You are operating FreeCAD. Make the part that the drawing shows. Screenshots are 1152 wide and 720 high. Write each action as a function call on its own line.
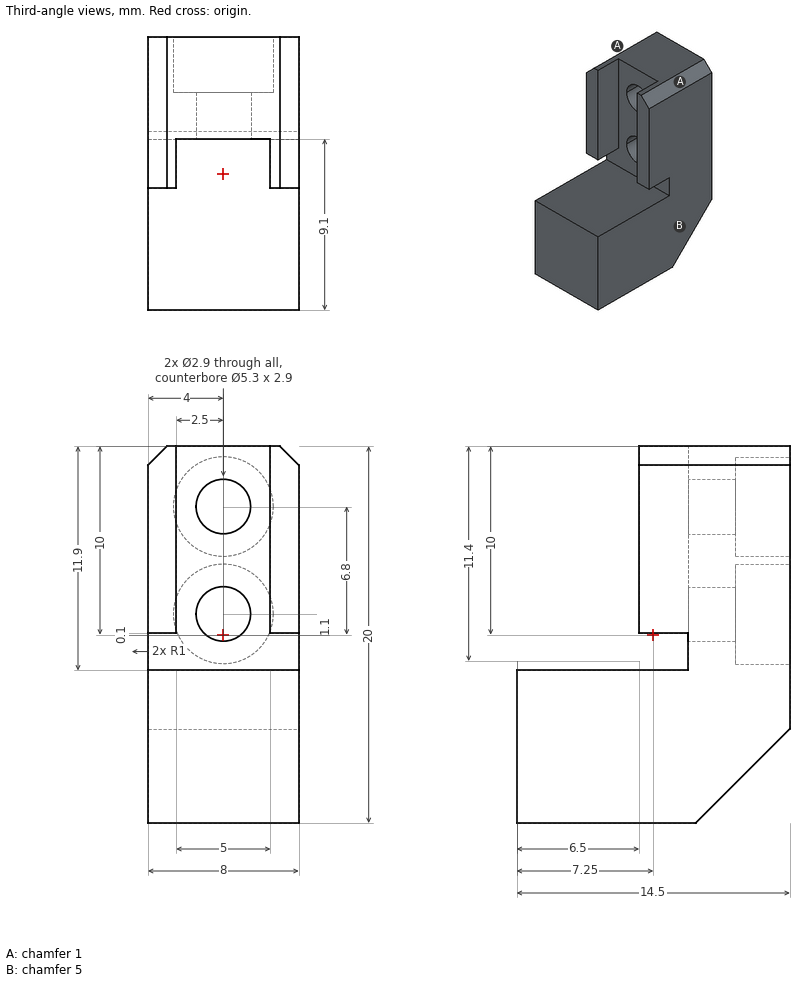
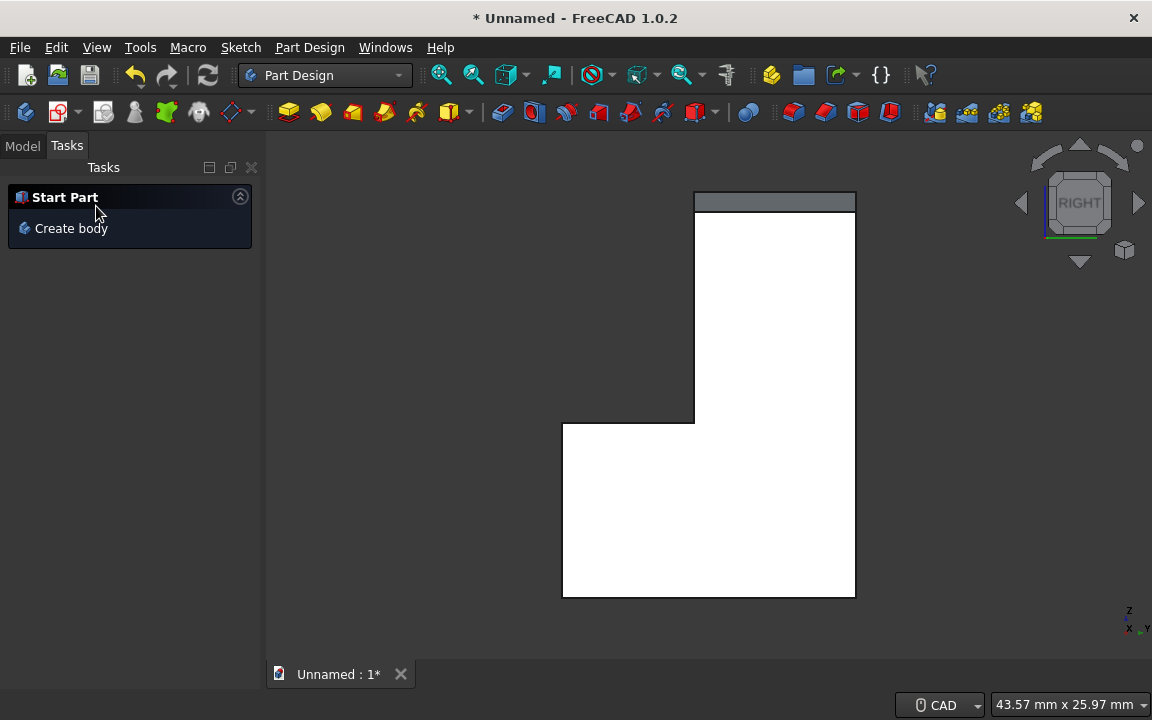
key(5)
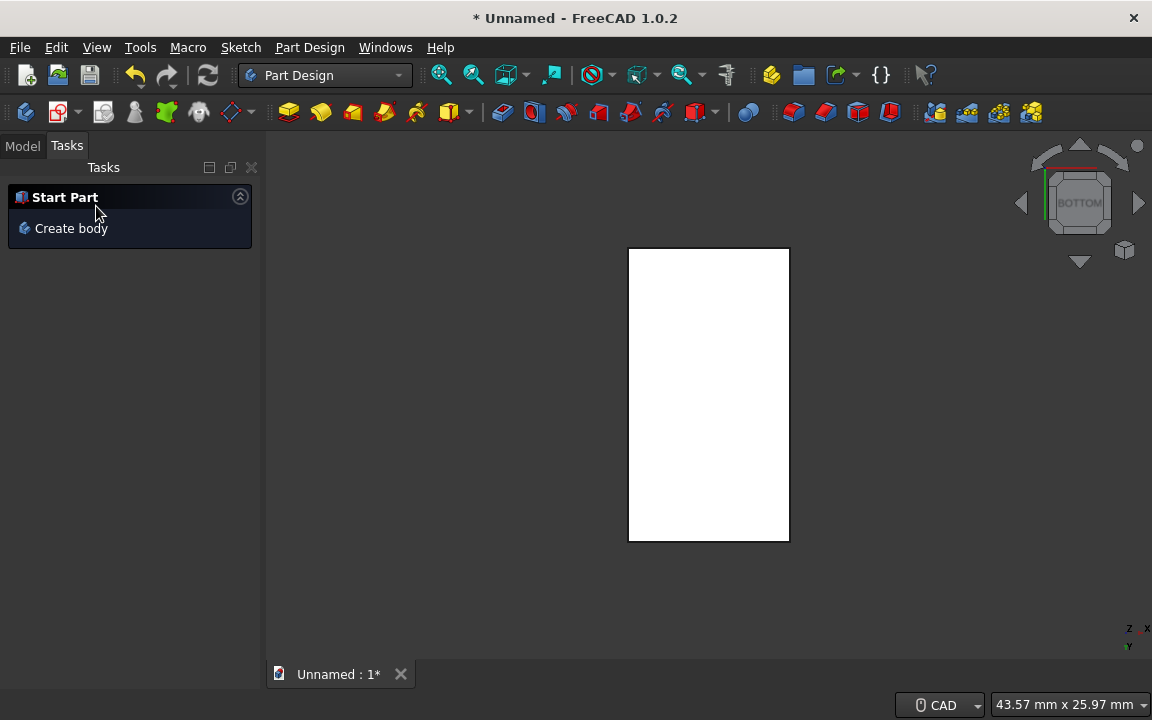
key(4)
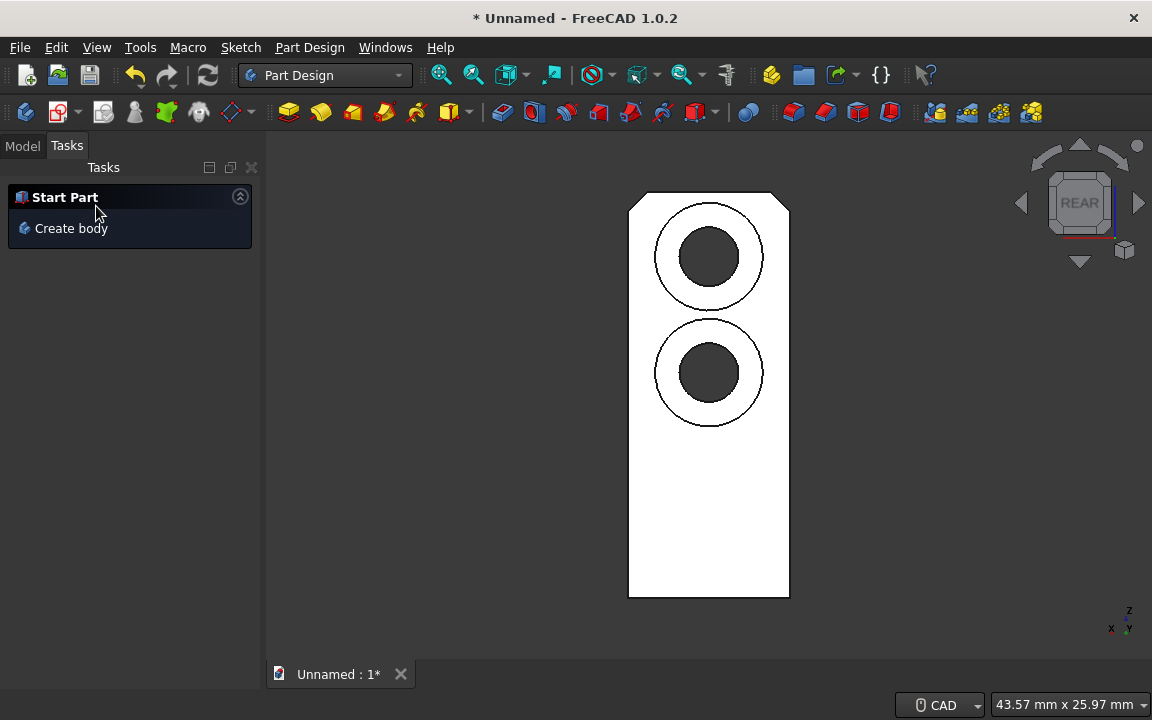
click(709, 597)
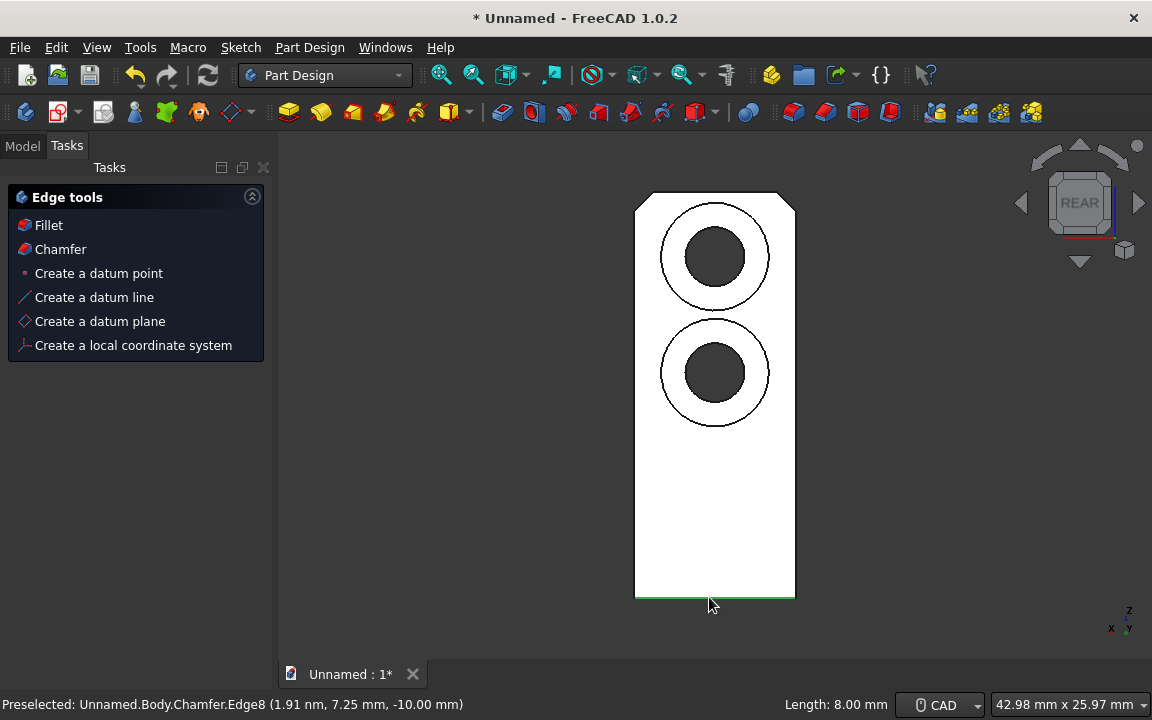
click(826, 112)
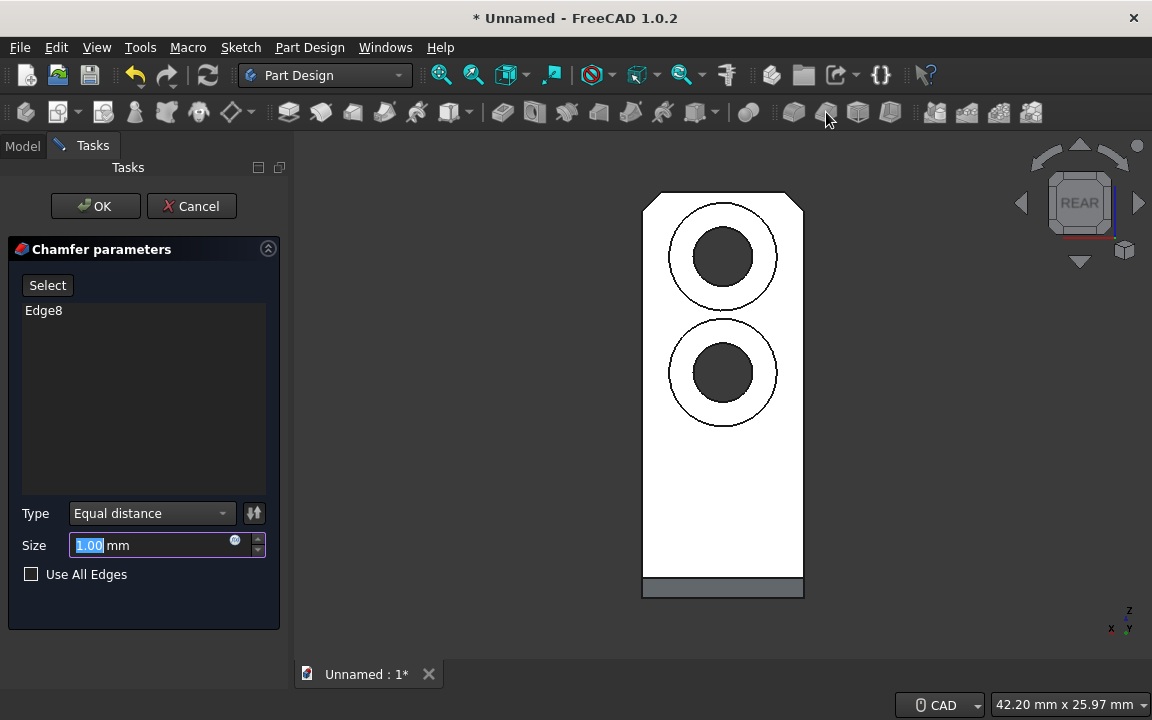
text(5)
key(Tab)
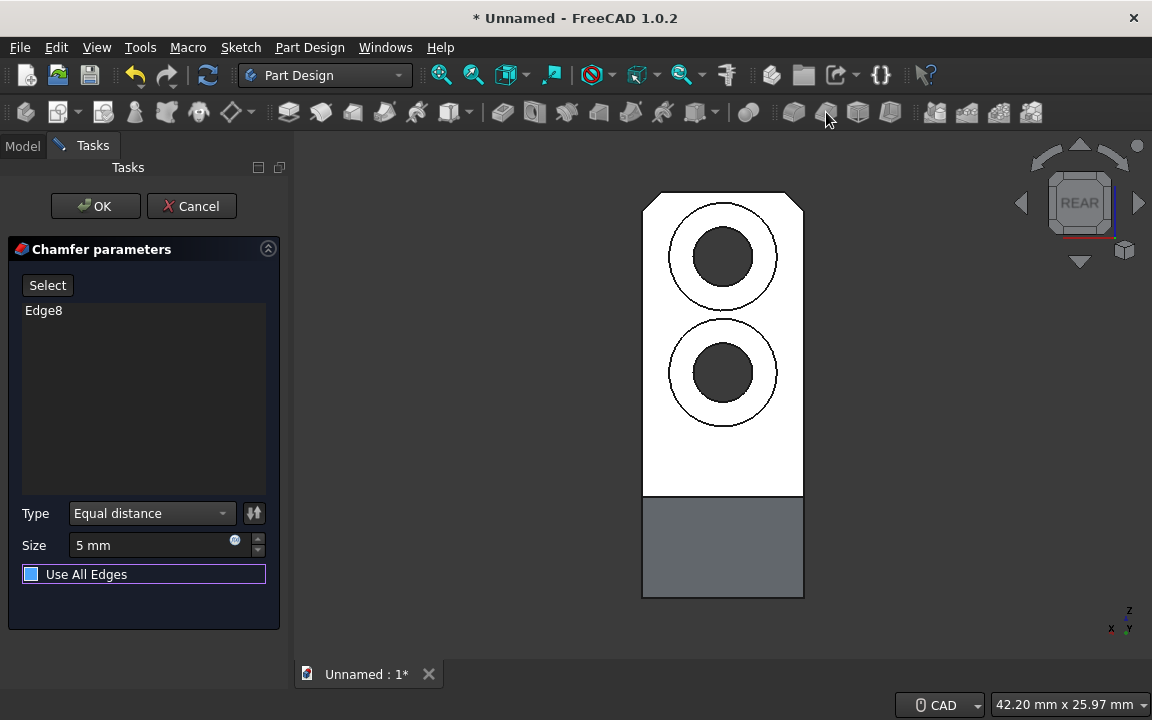
click(96, 206)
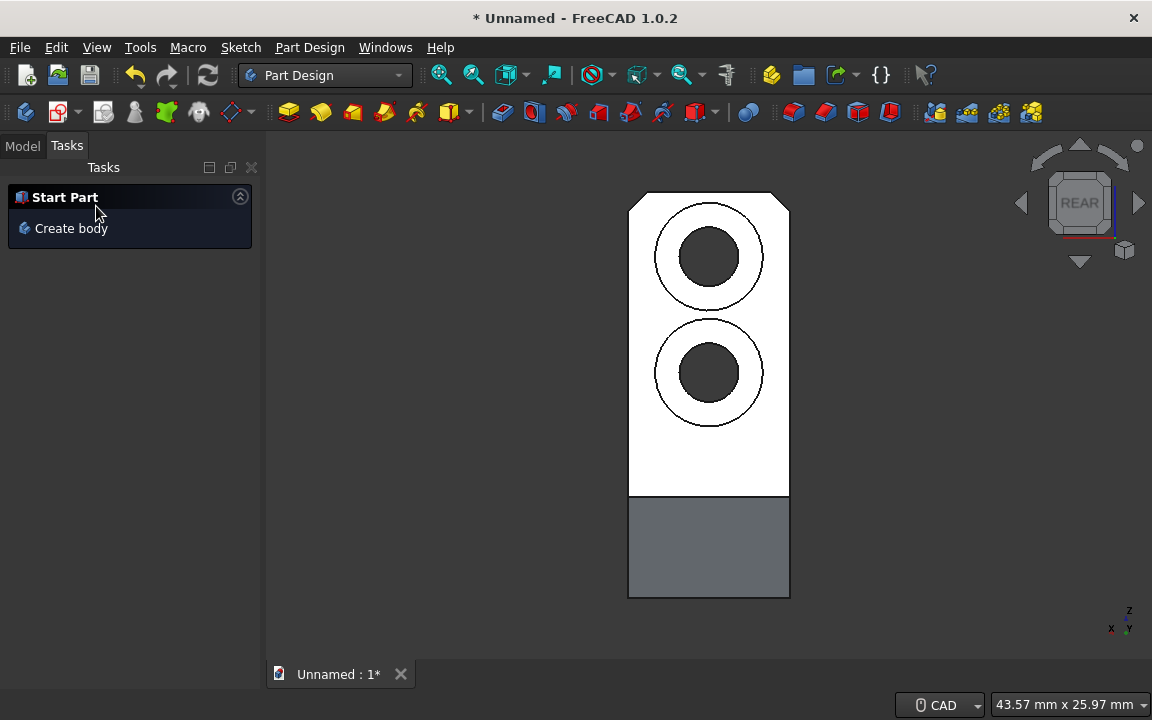
key(0)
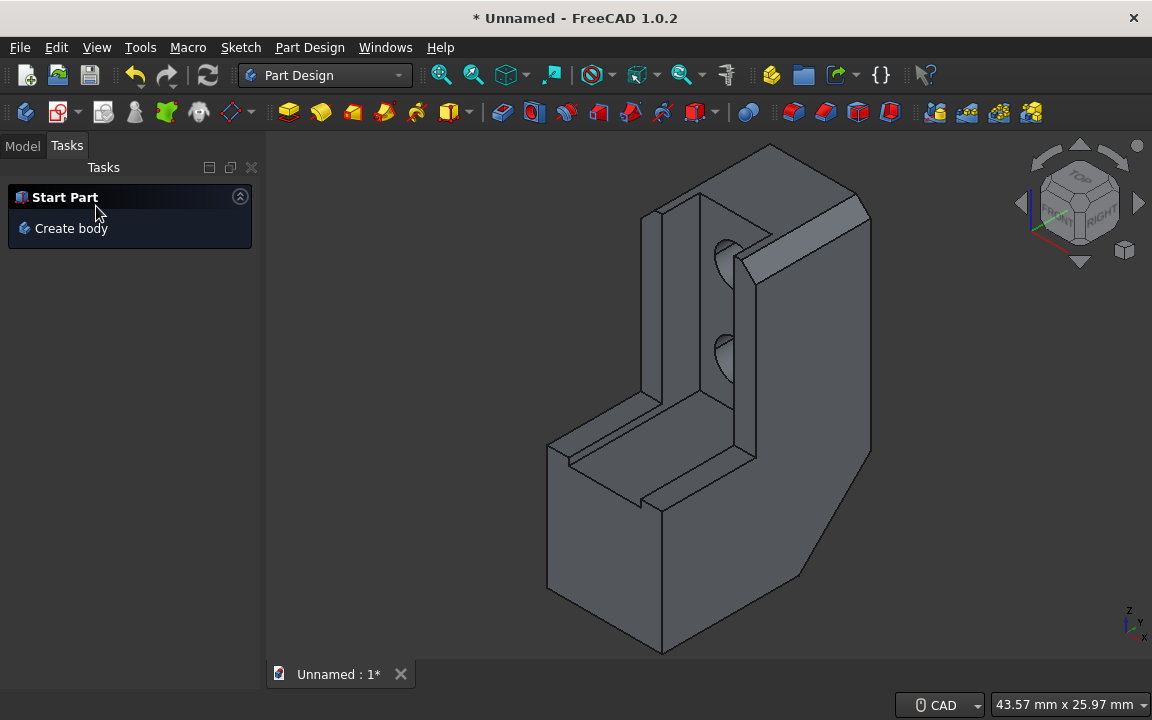
click(605, 549)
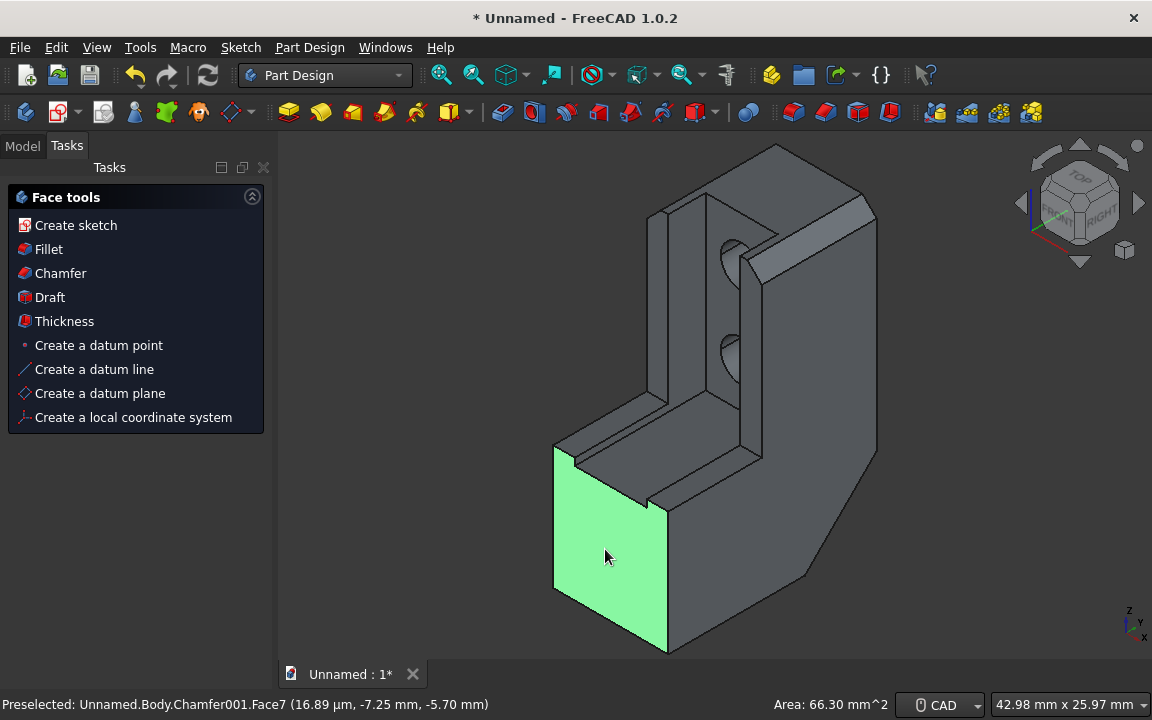
click(58, 112)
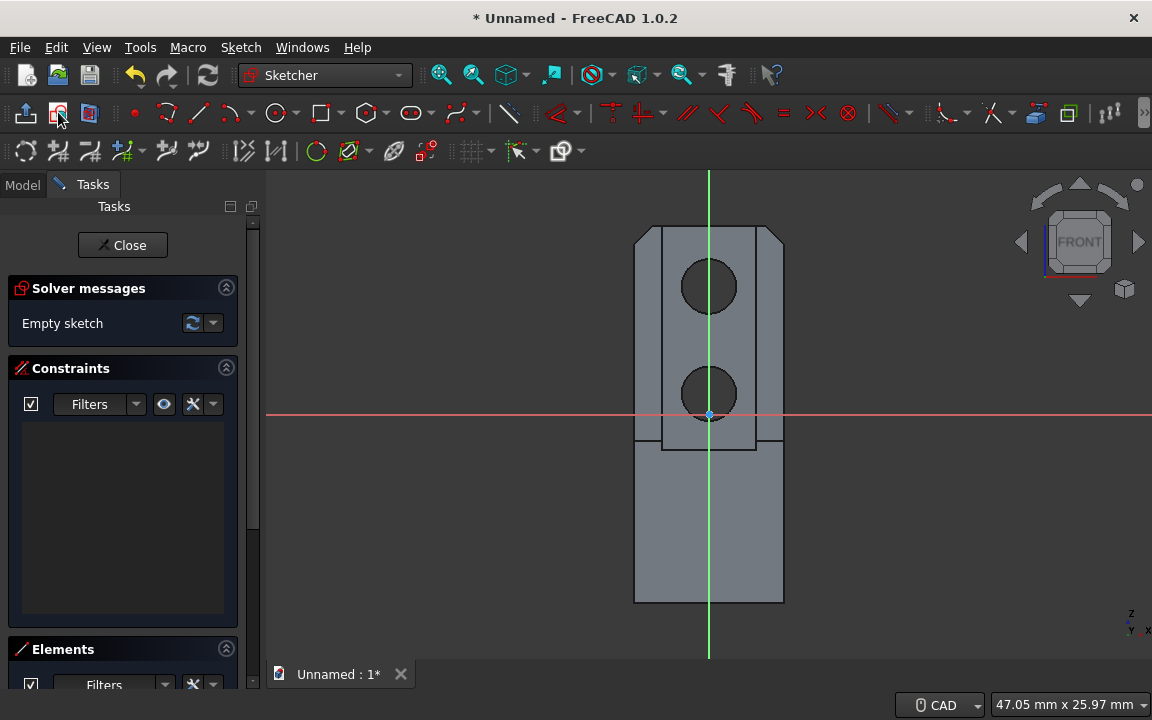
scroll(749, 441, up, 5)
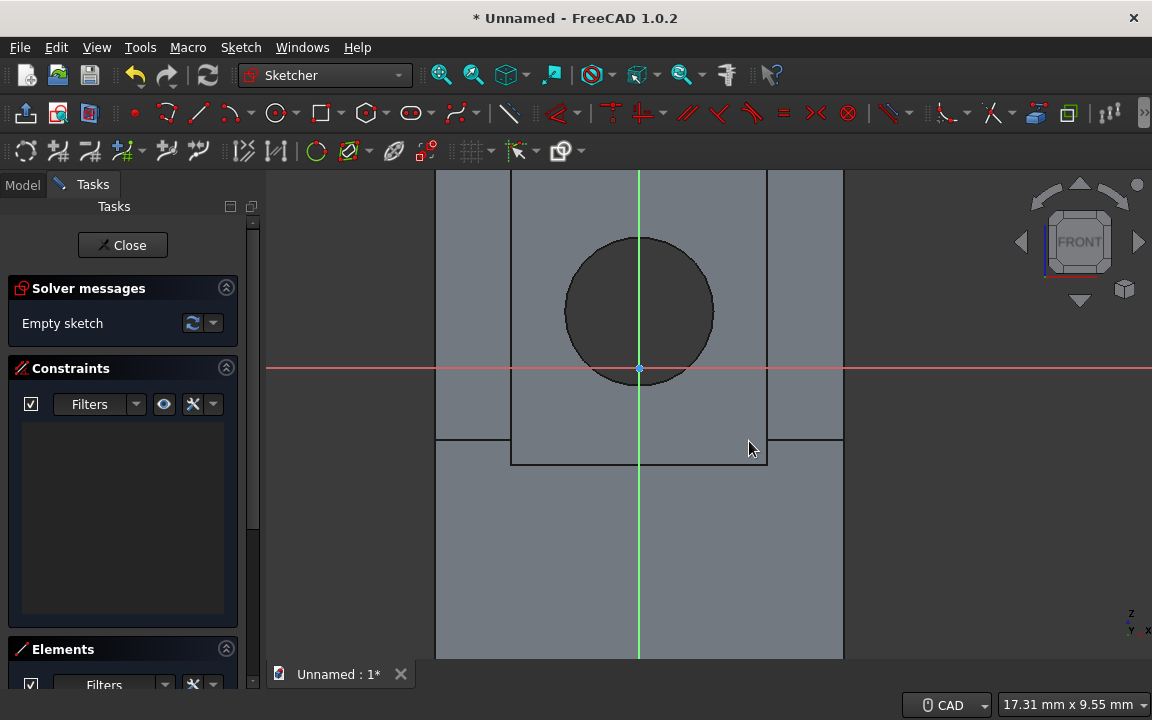
key(g)
key(s)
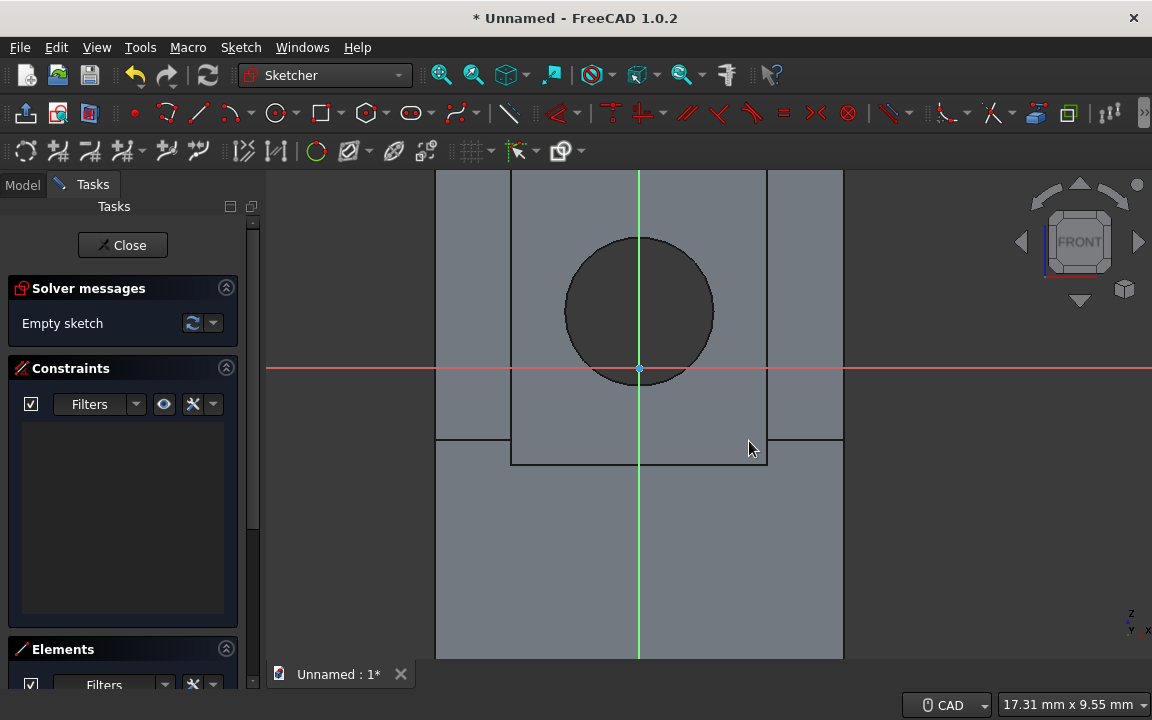
click(435, 414)